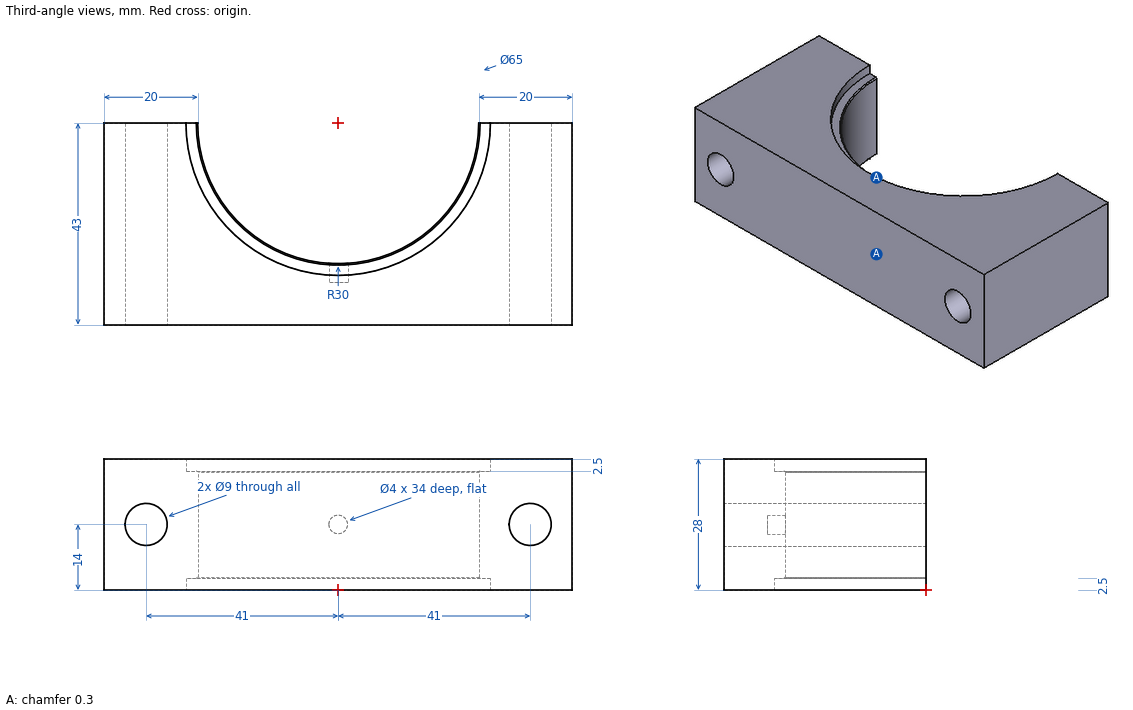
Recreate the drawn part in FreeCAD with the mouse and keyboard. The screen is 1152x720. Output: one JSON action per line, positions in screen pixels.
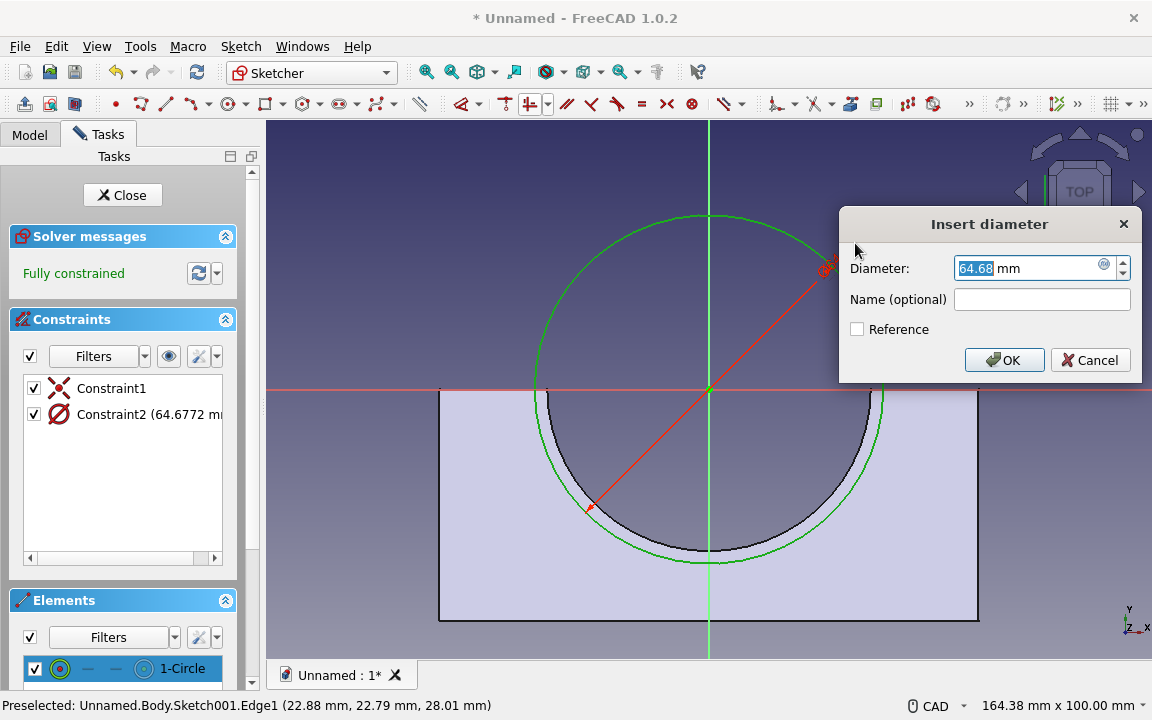
{"action": "type", "text": "65"}
{"action": "key", "text": "Return"}
{"action": "key", "text": "Escape"}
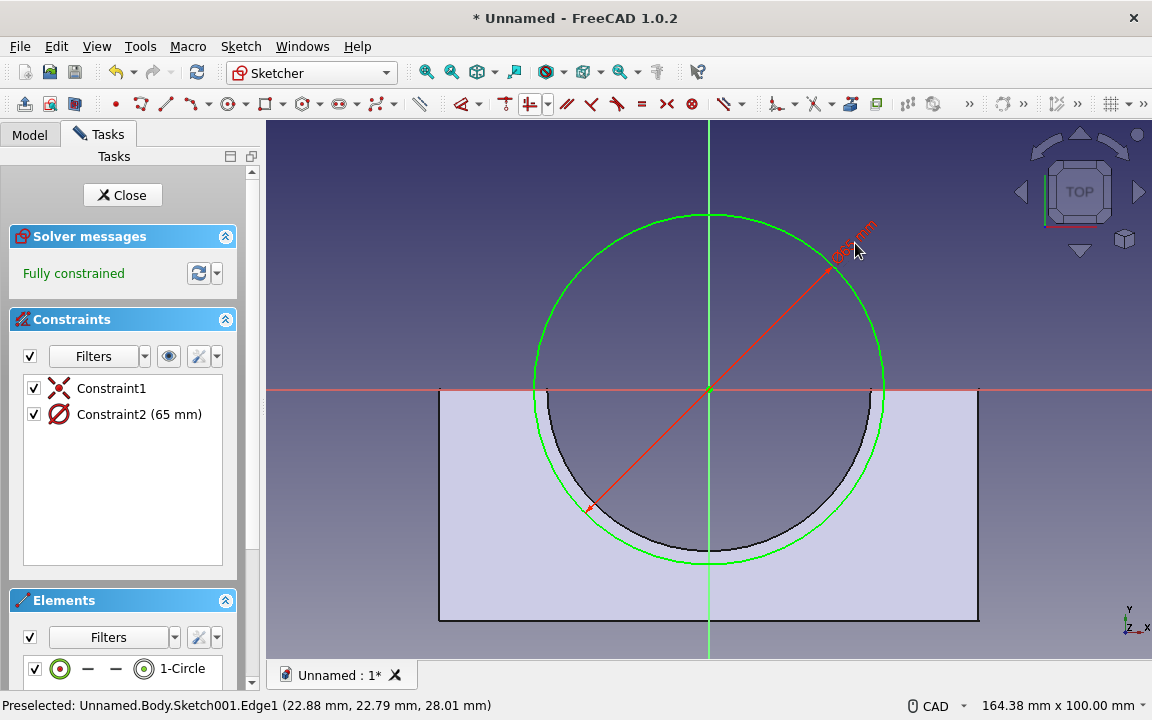
{"action": "left_click", "coordinate": [123, 195]}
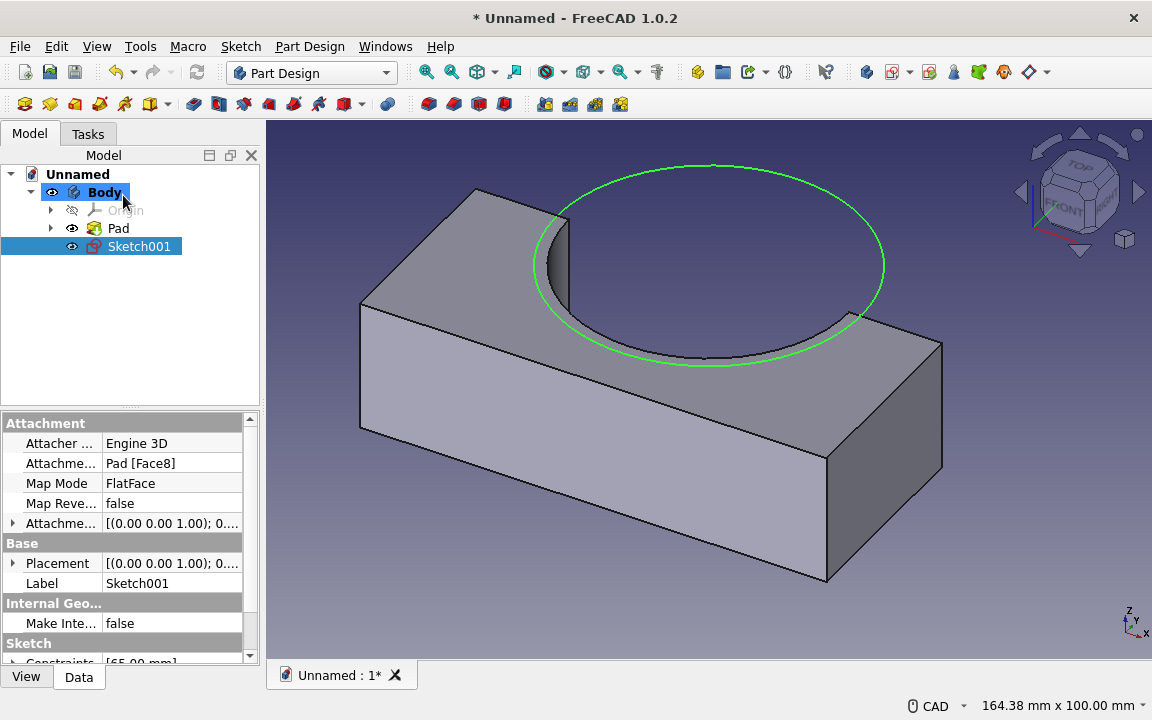
{"action": "left_click", "coordinate": [194, 104]}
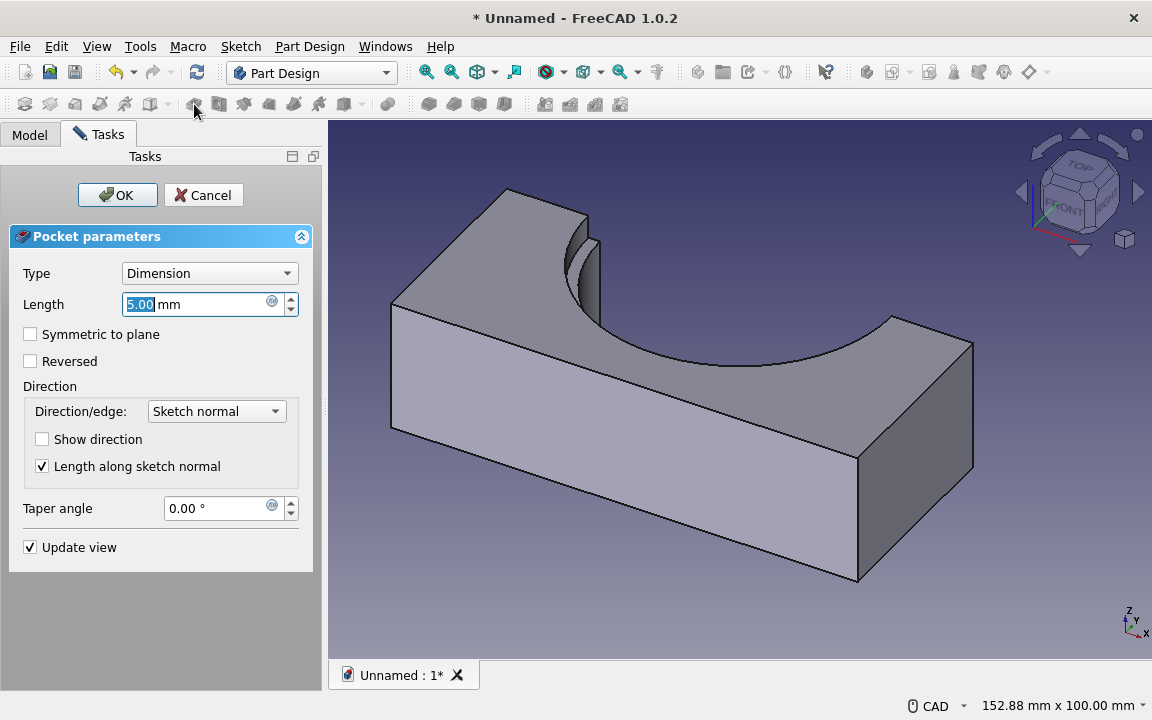
{"action": "type", "text": "2.5"}
{"action": "key", "text": "Tab"}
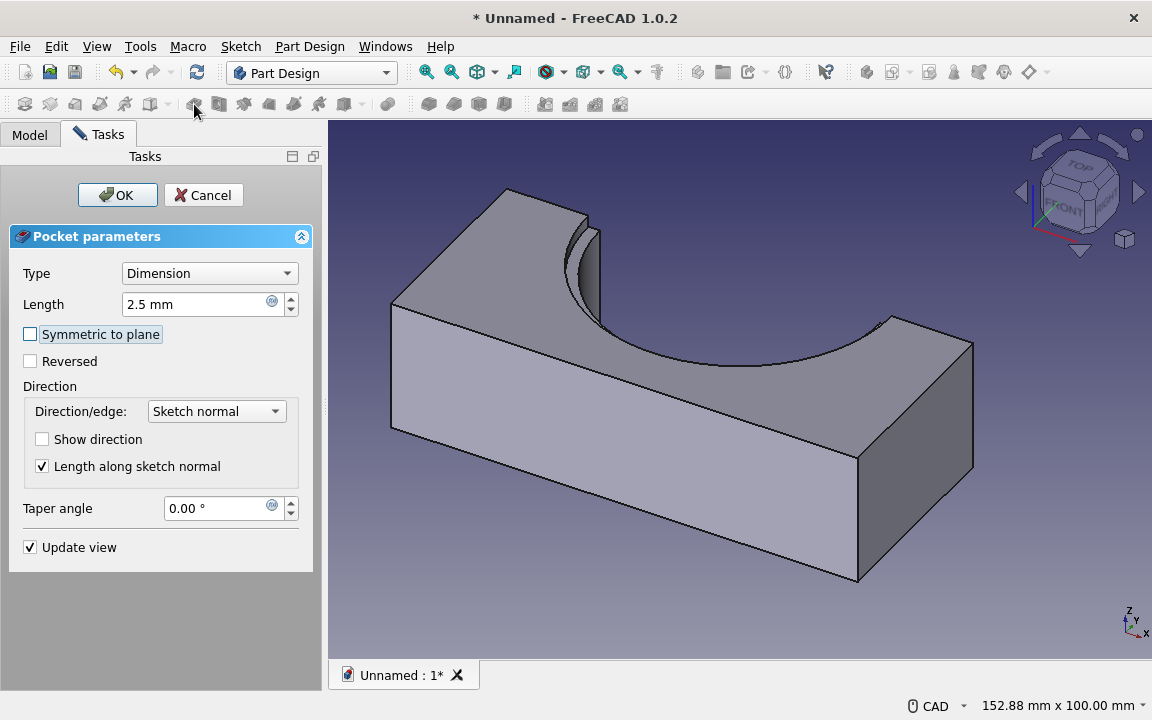
{"action": "left_click", "coordinate": [118, 195]}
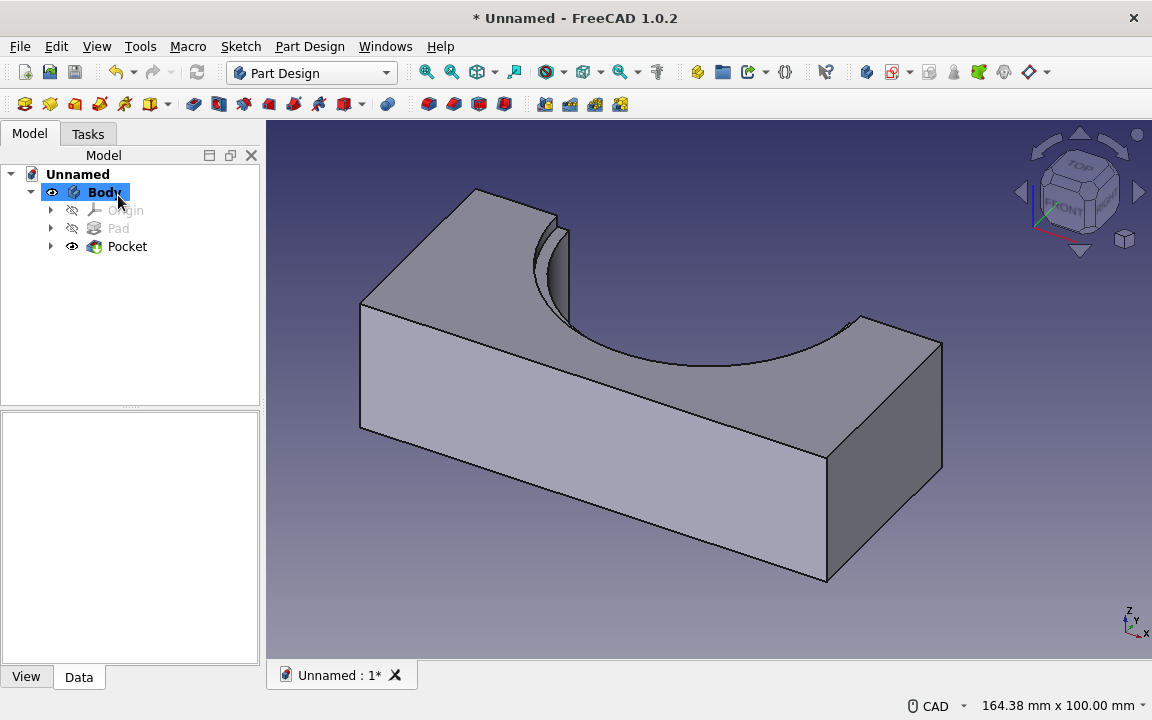
{"action": "left_click", "coordinate": [51, 210]}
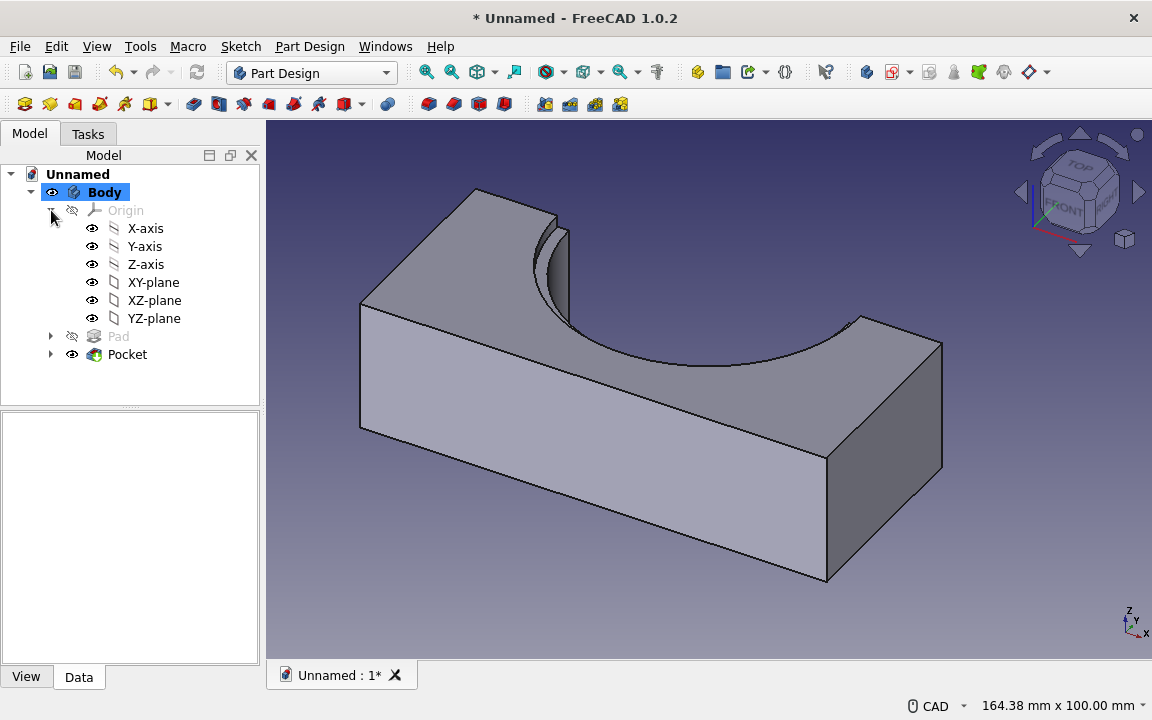
{"action": "left_click", "coordinate": [137, 282]}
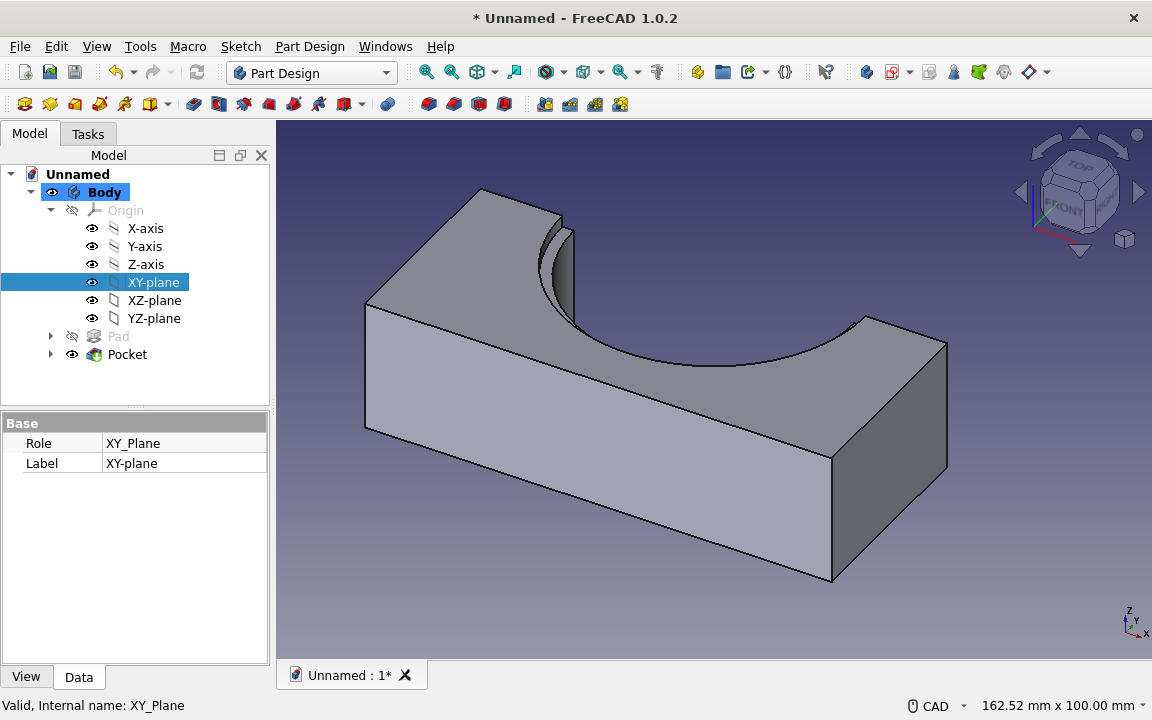
{"action": "left_click", "coordinate": [1028, 72]}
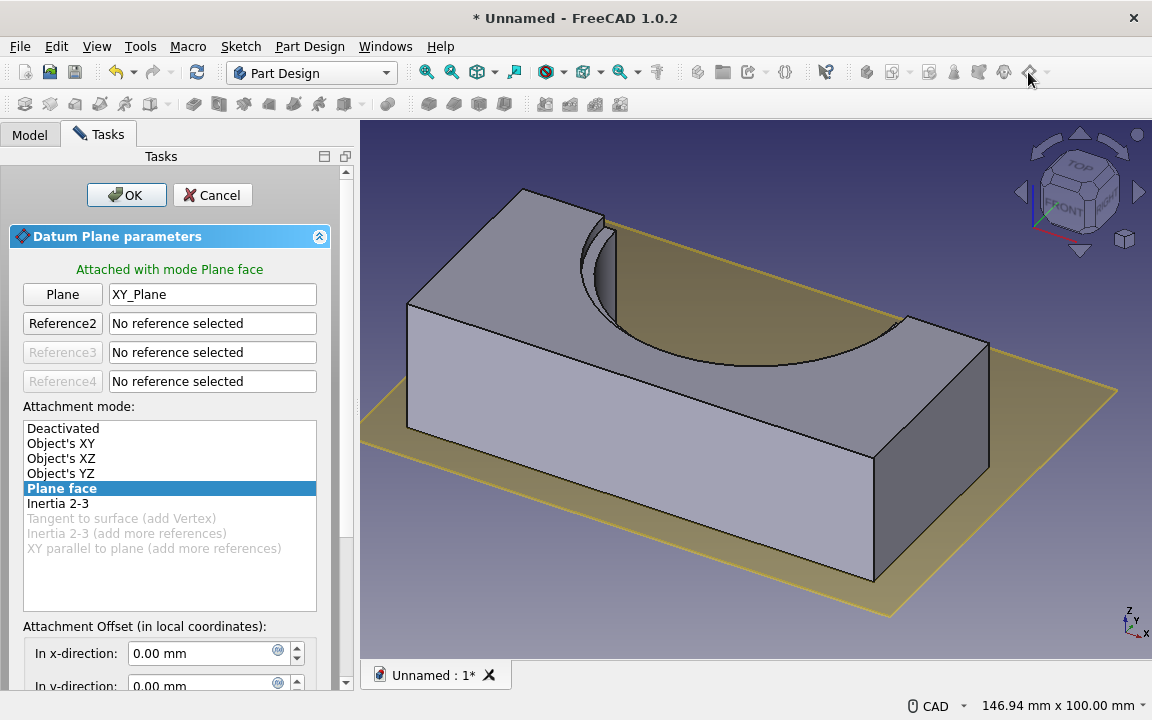
{"action": "scroll", "coordinate": [346, 428], "scroll_direction": "down", "scroll_amount": 2}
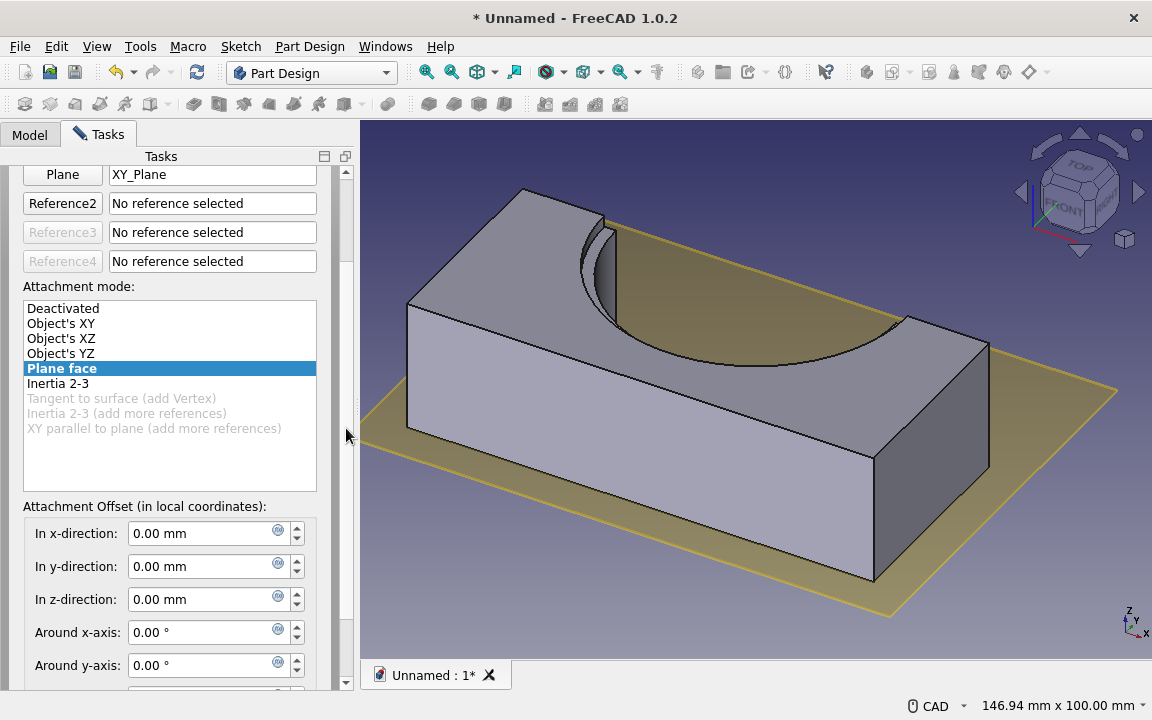
{"action": "triple_click", "coordinate": [210, 600]}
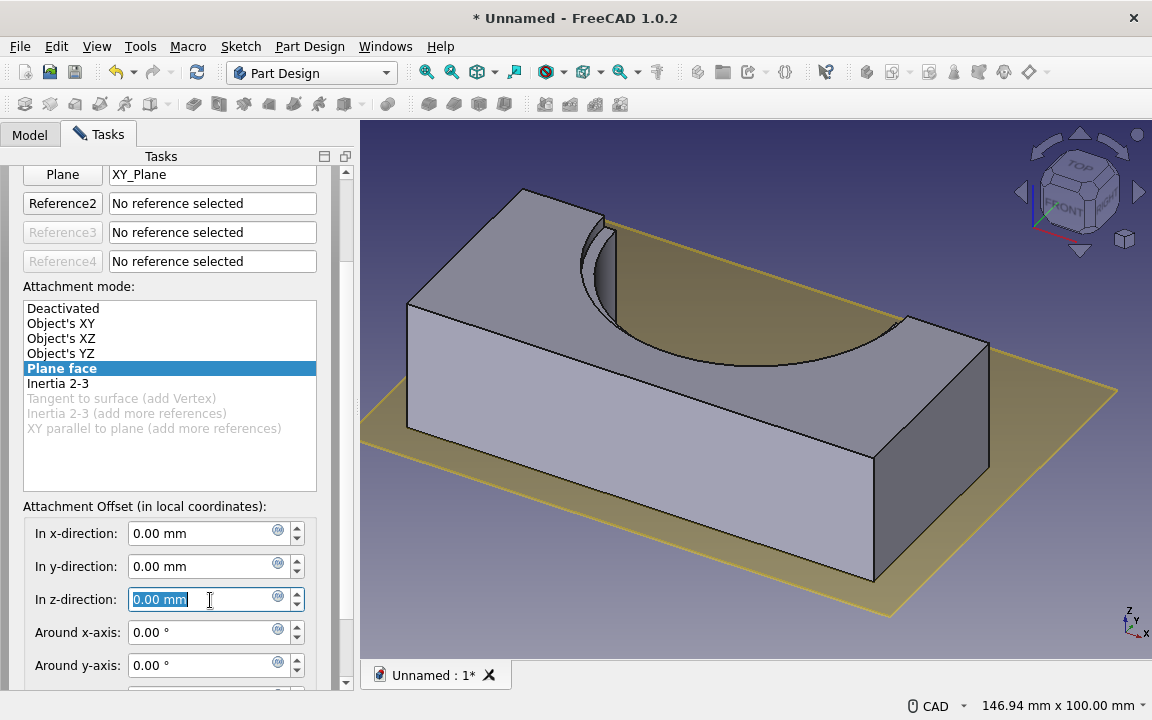
{"action": "type", "text": "2.5"}
{"action": "key", "text": "Tab"}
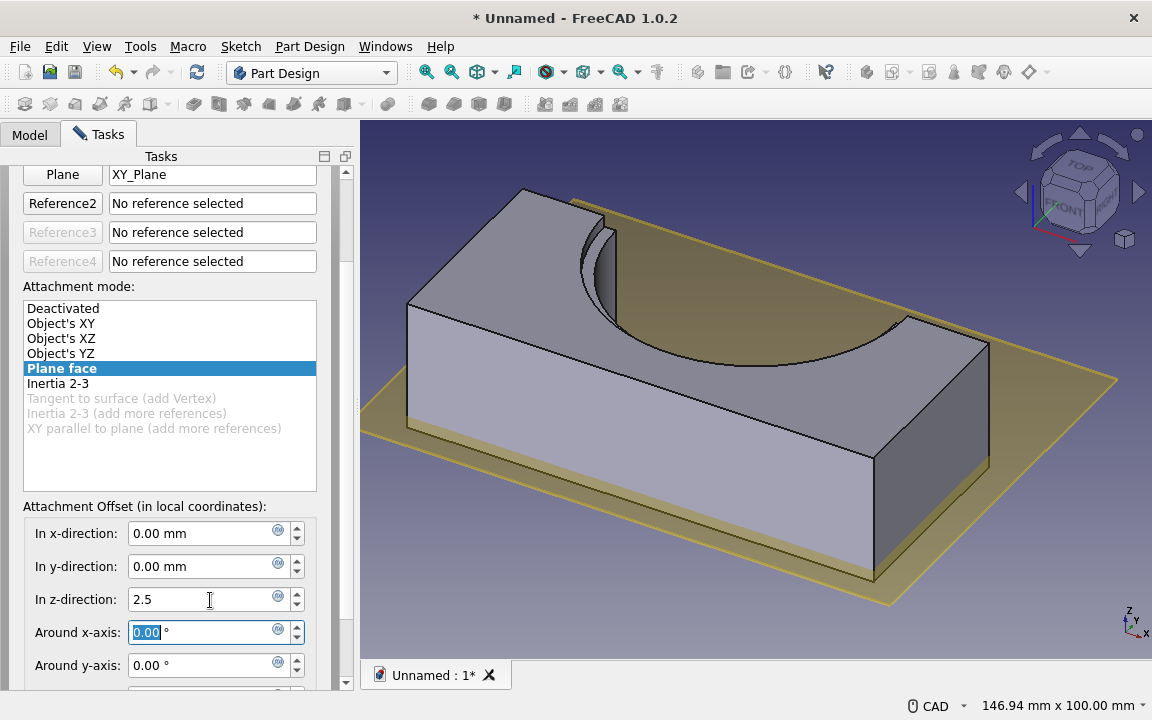
{"action": "scroll", "coordinate": [346, 428], "scroll_direction": "up", "scroll_amount": 3}